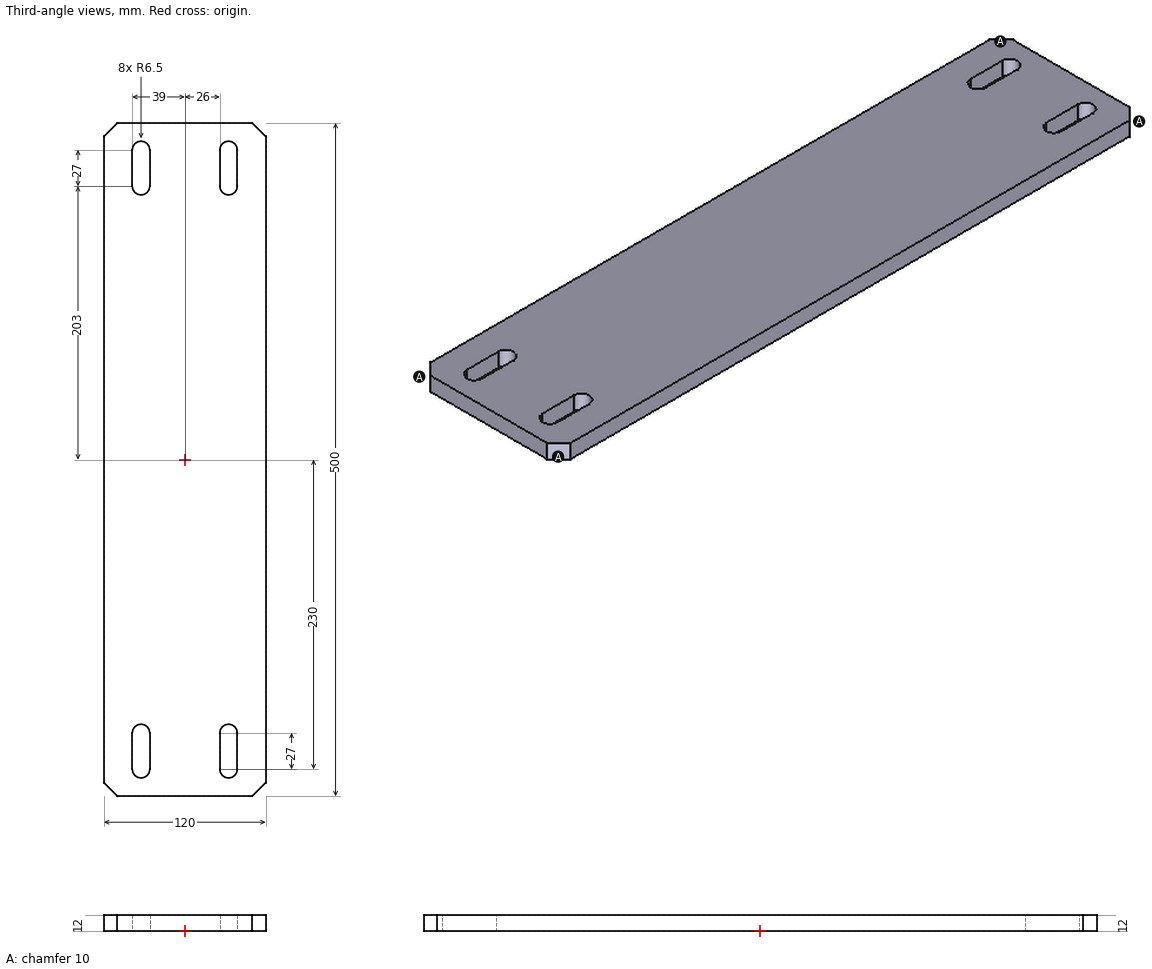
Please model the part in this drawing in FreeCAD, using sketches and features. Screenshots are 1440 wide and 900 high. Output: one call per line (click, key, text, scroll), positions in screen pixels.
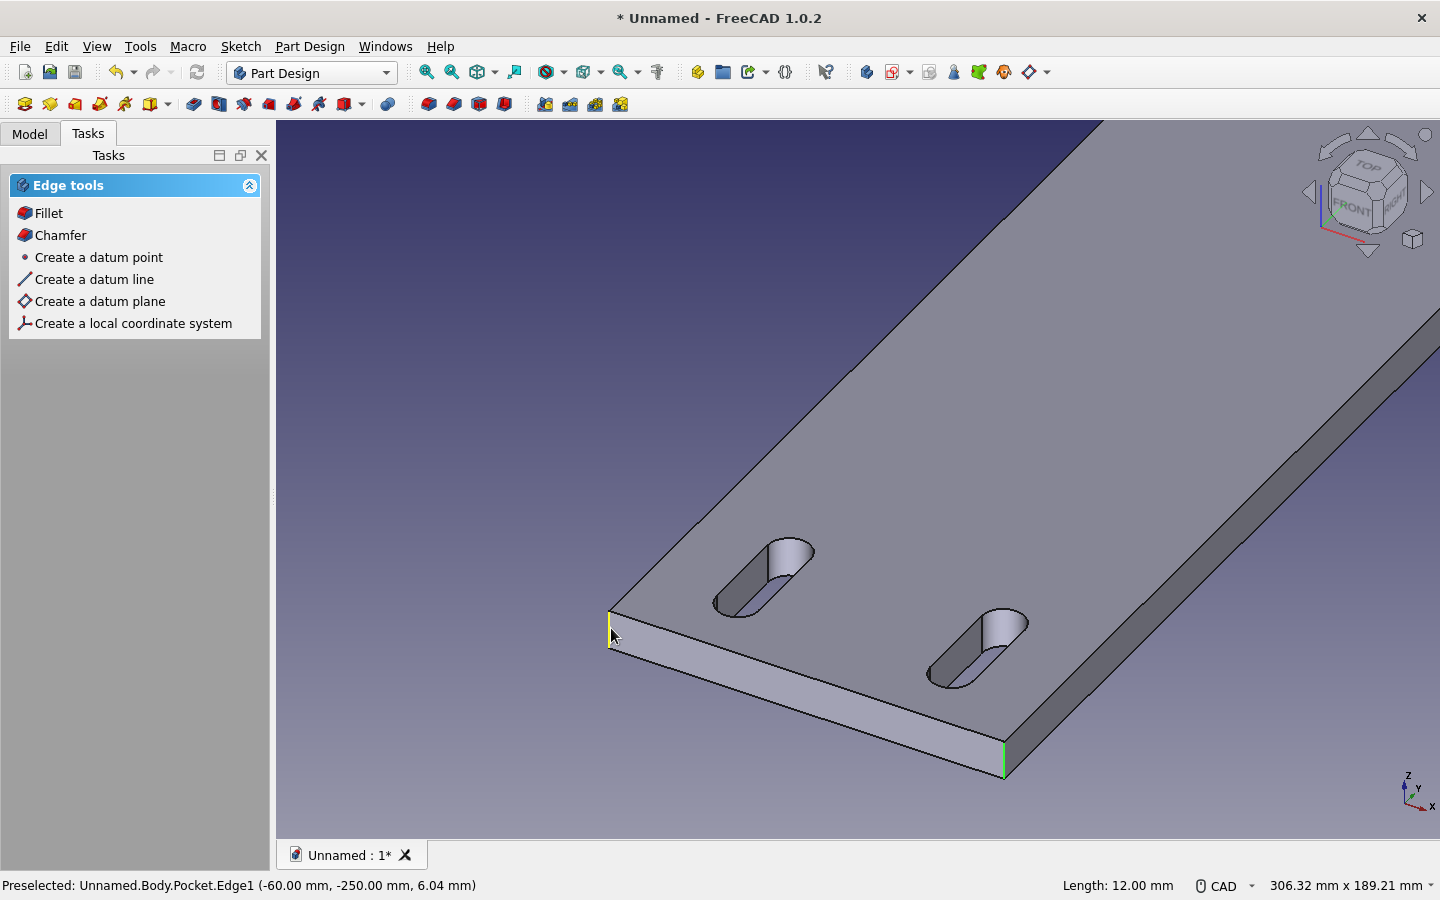
key(v)
key(f)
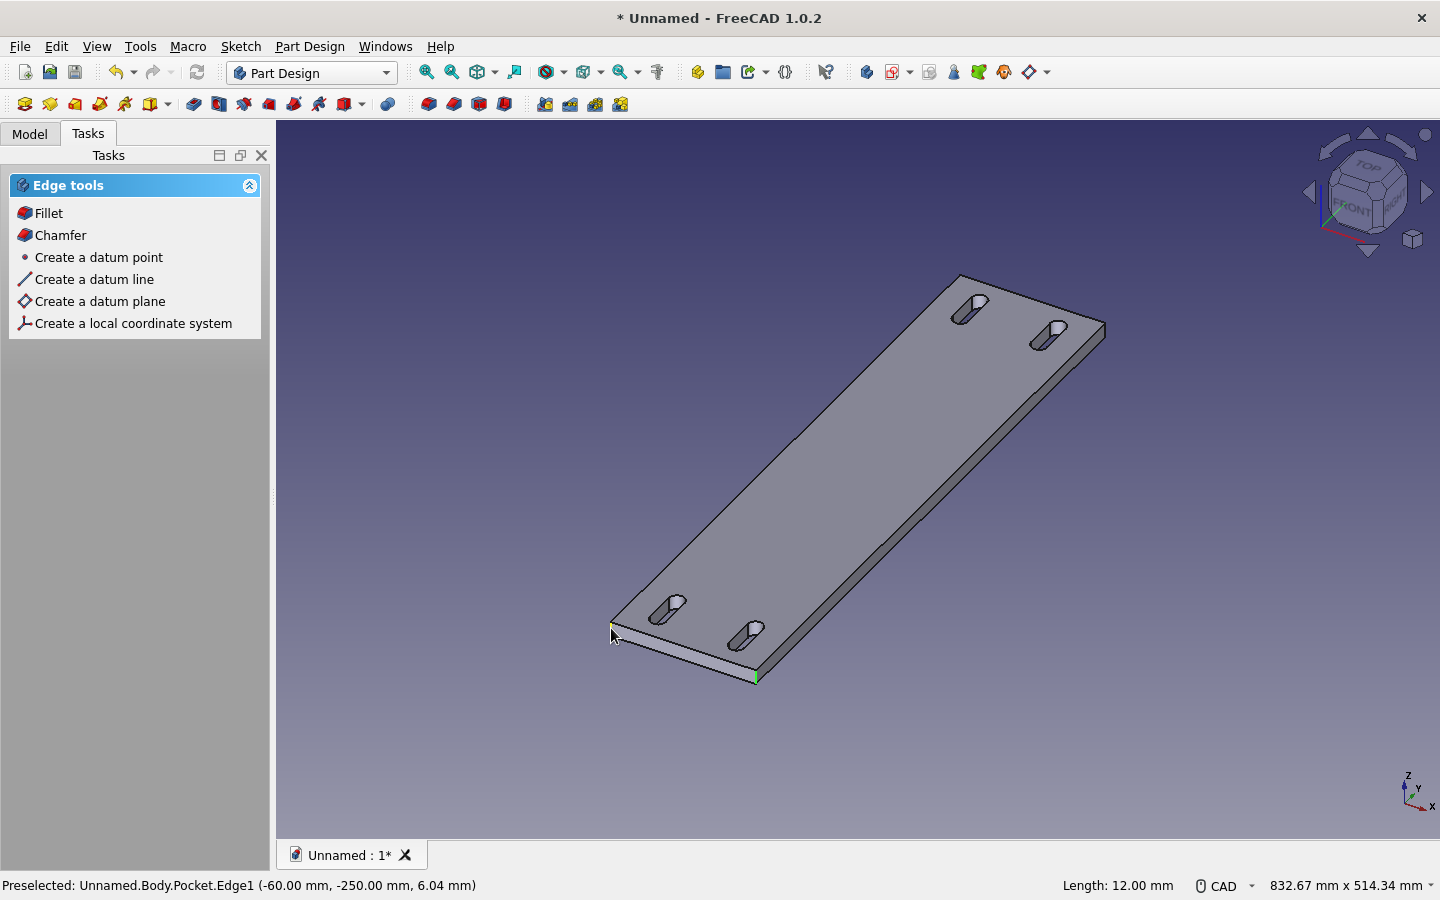
key(0)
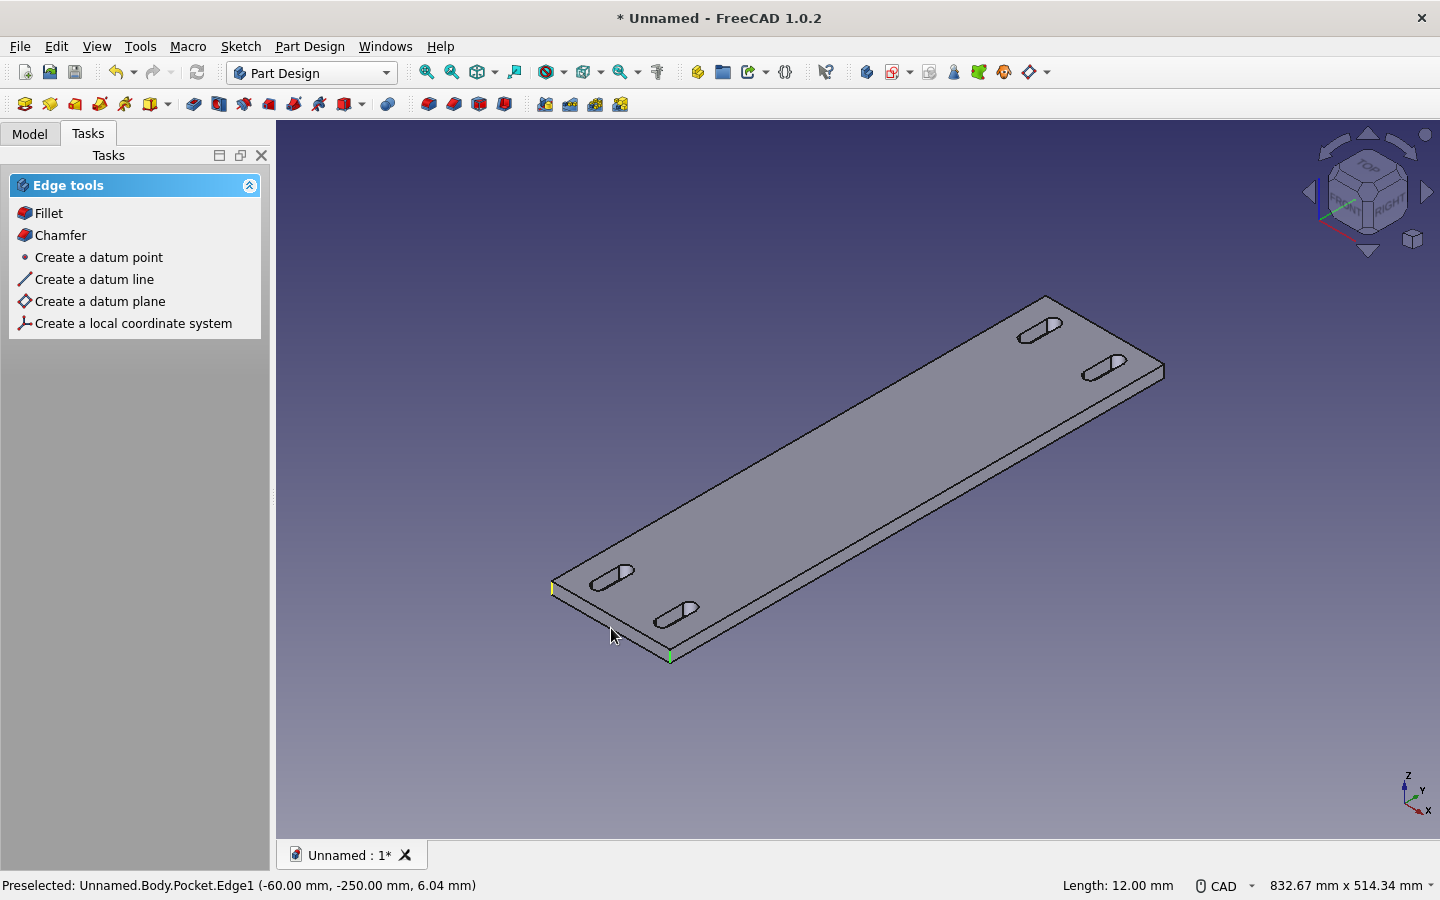
scroll(552, 587, up, 5)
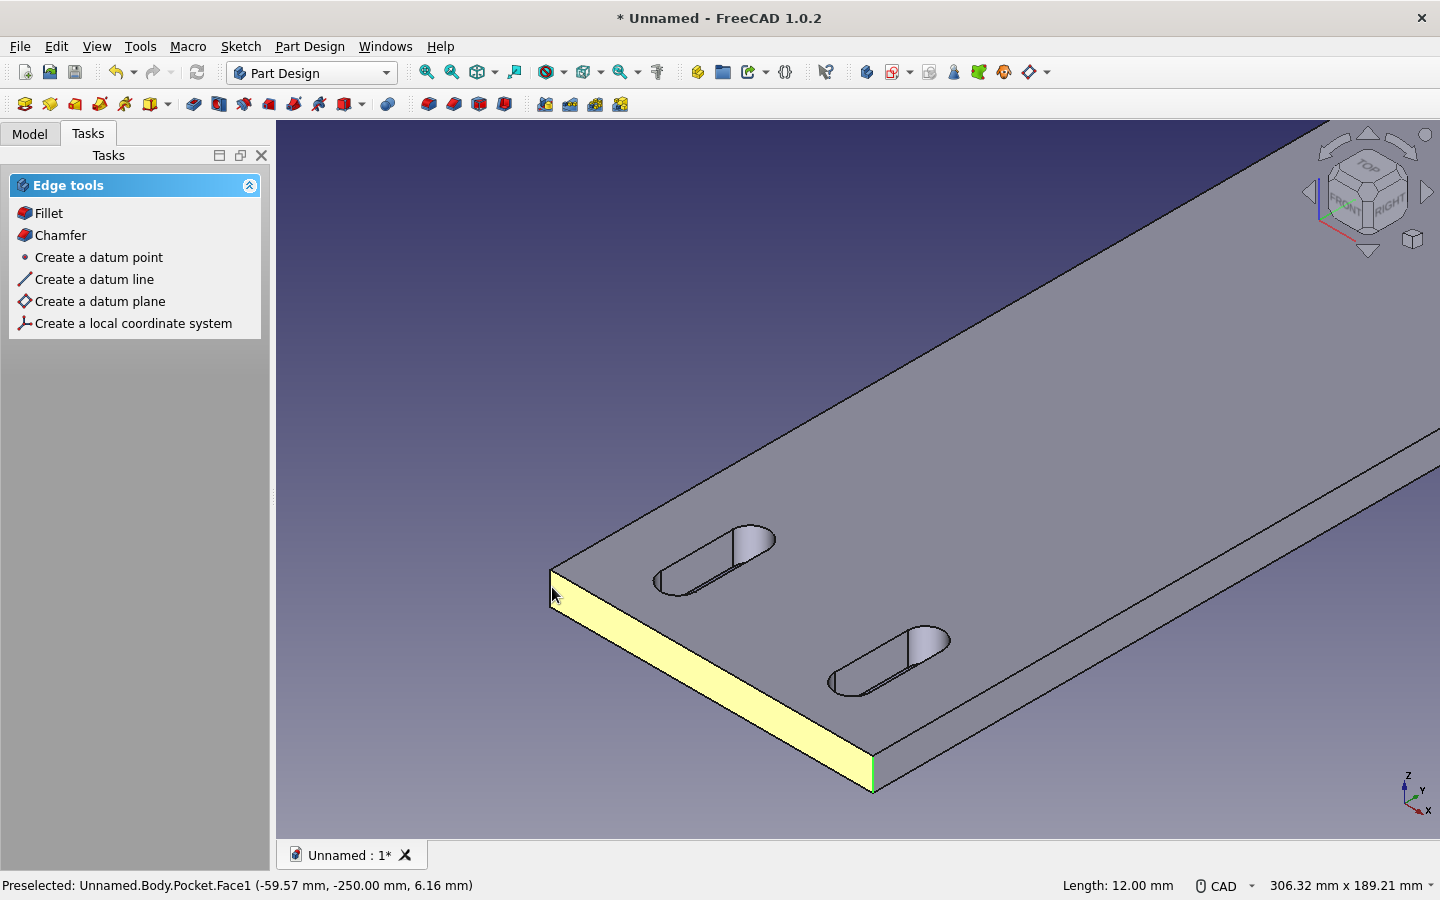
key(v)
key(f)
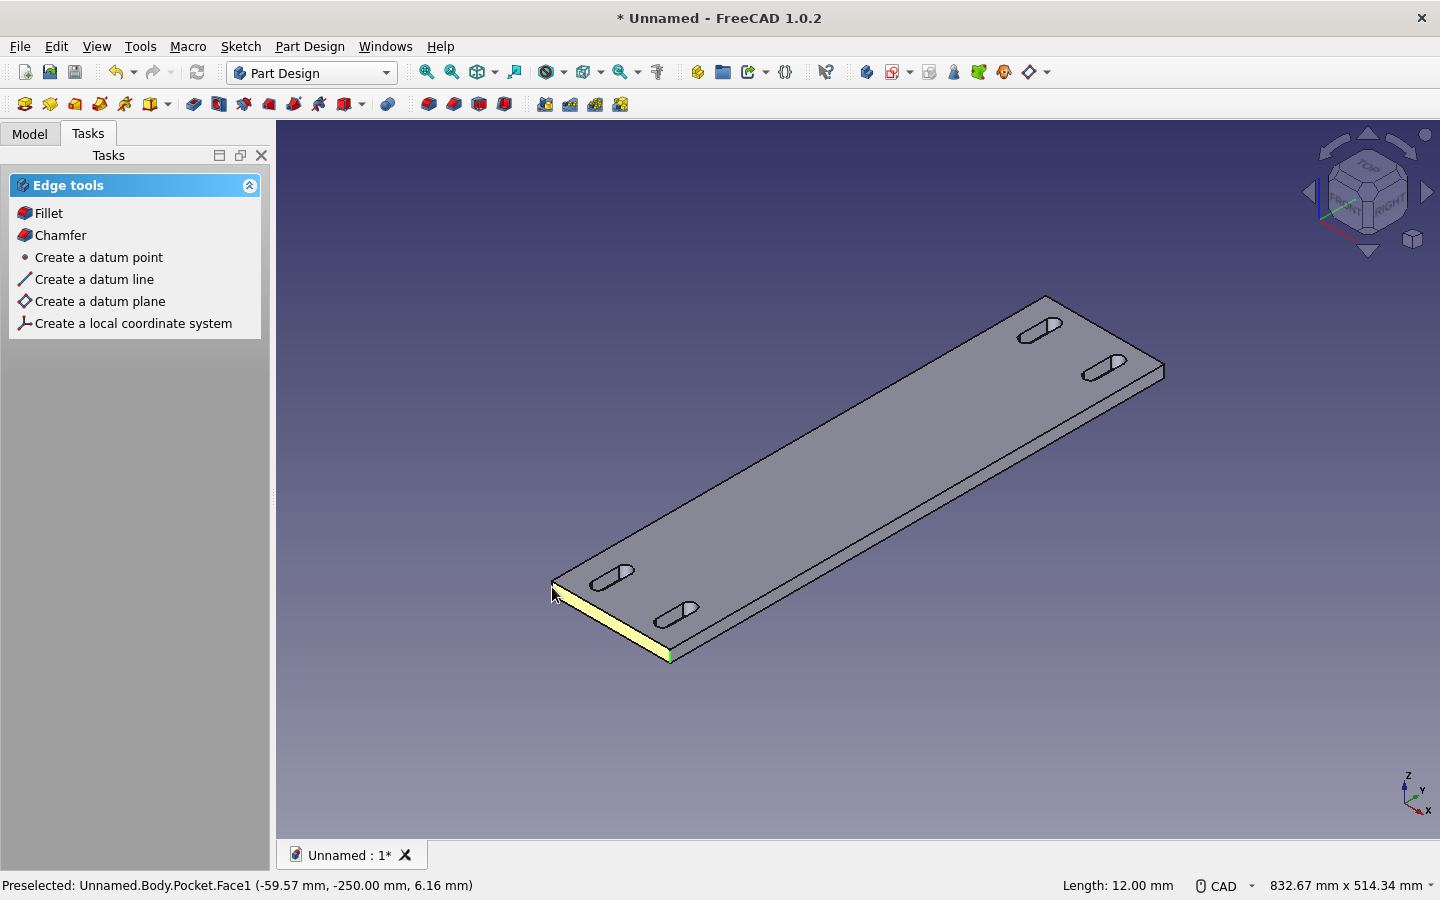
key(2)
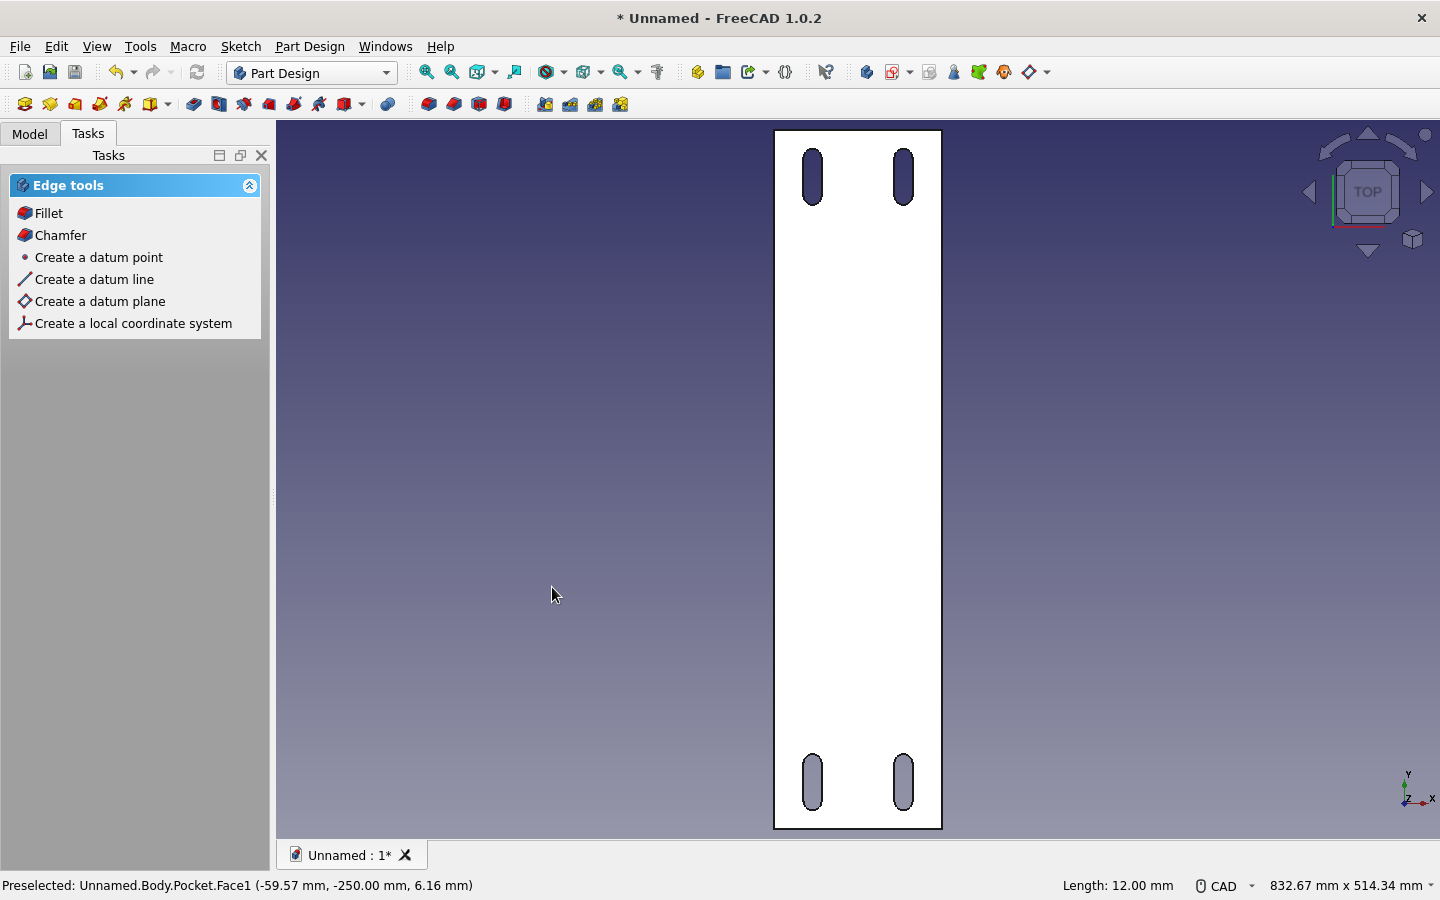
key(1)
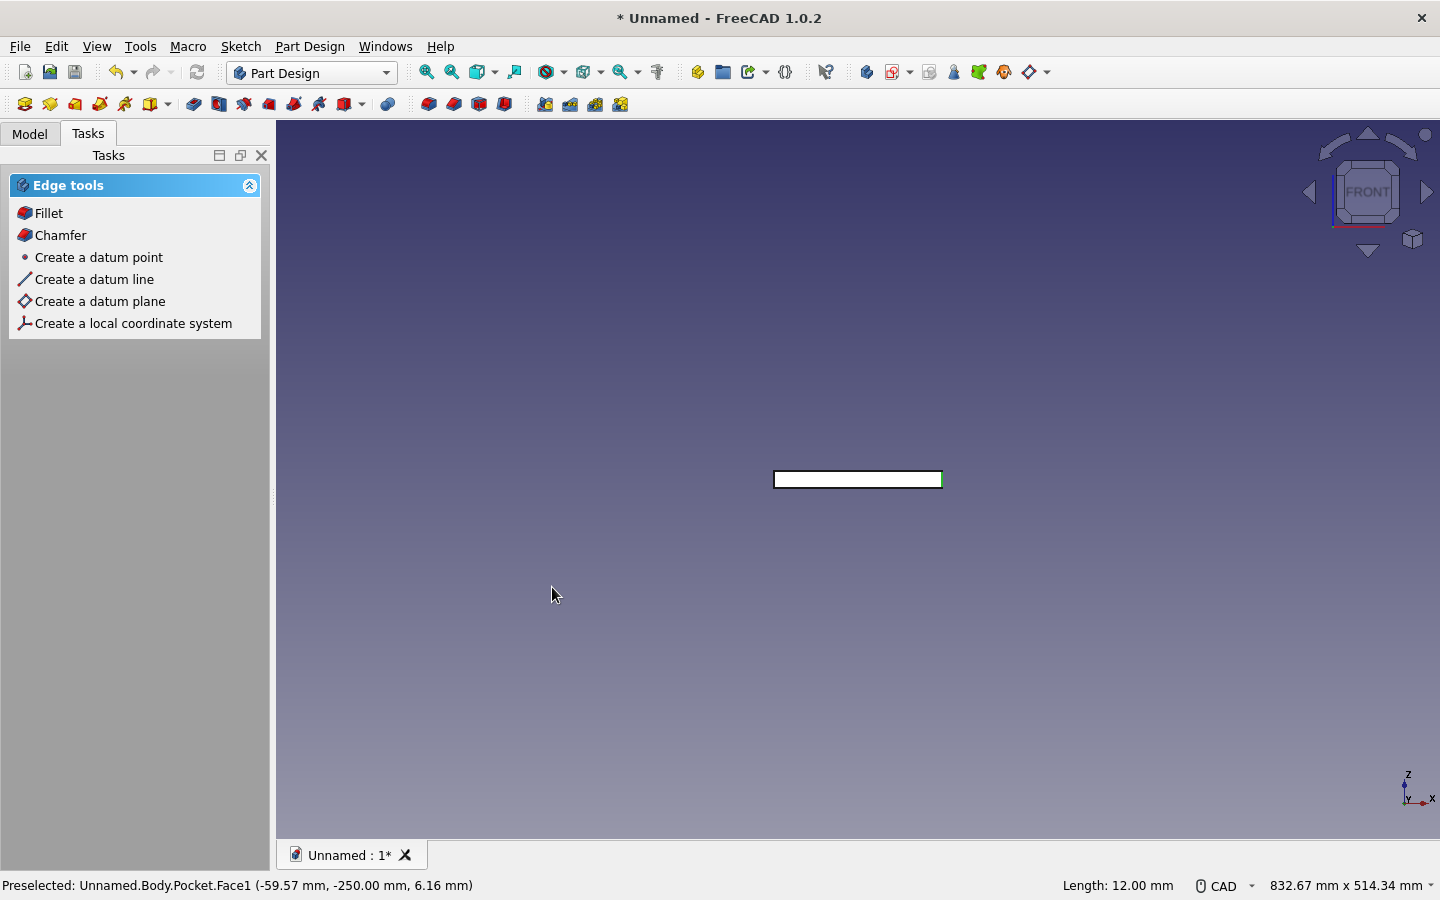
click(427, 72)